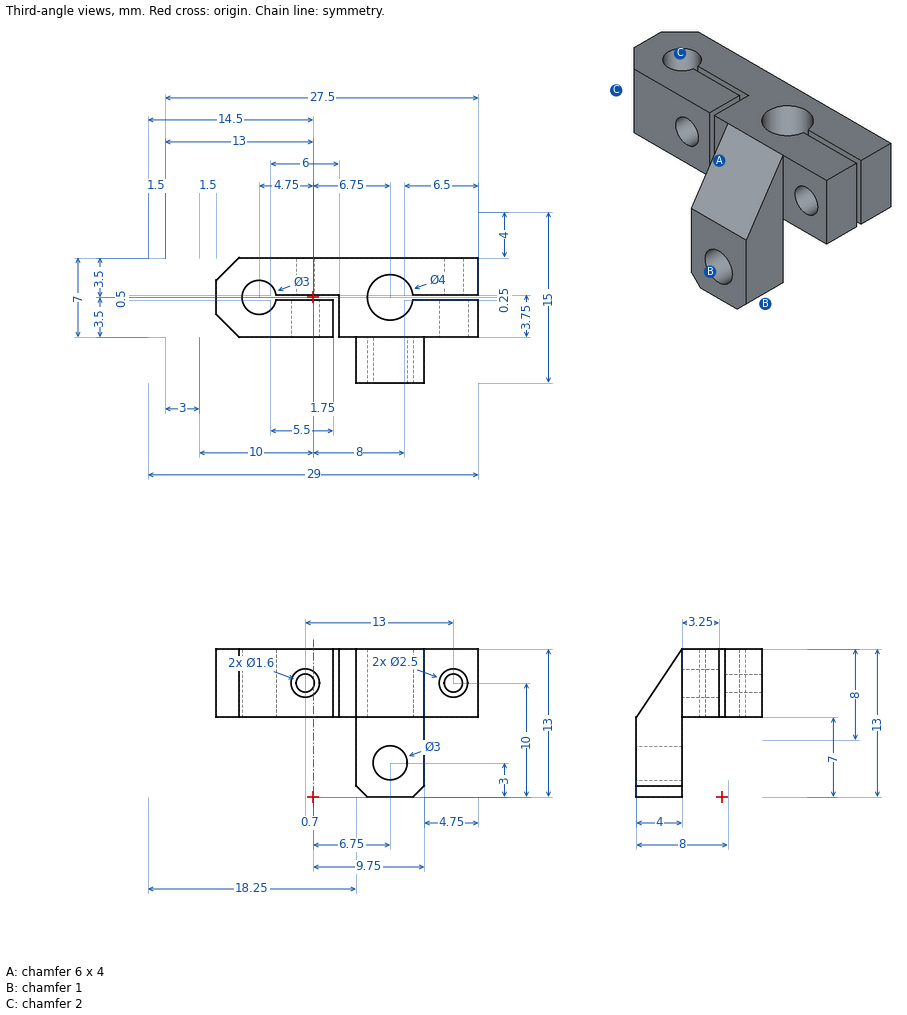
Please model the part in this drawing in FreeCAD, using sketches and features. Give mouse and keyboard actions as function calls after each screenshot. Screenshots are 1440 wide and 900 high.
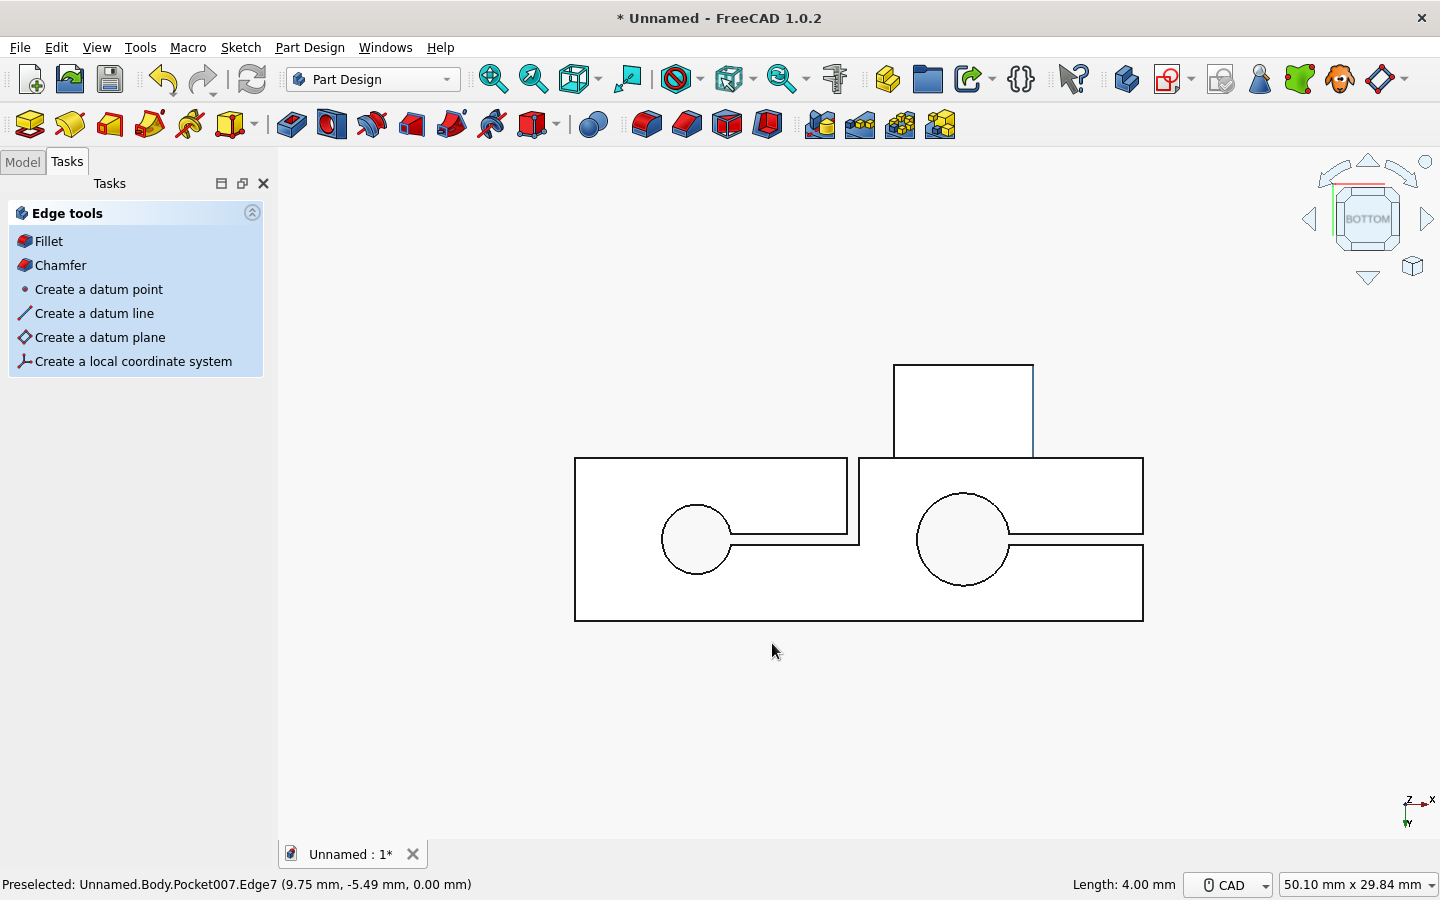
click(894, 392, ctrl)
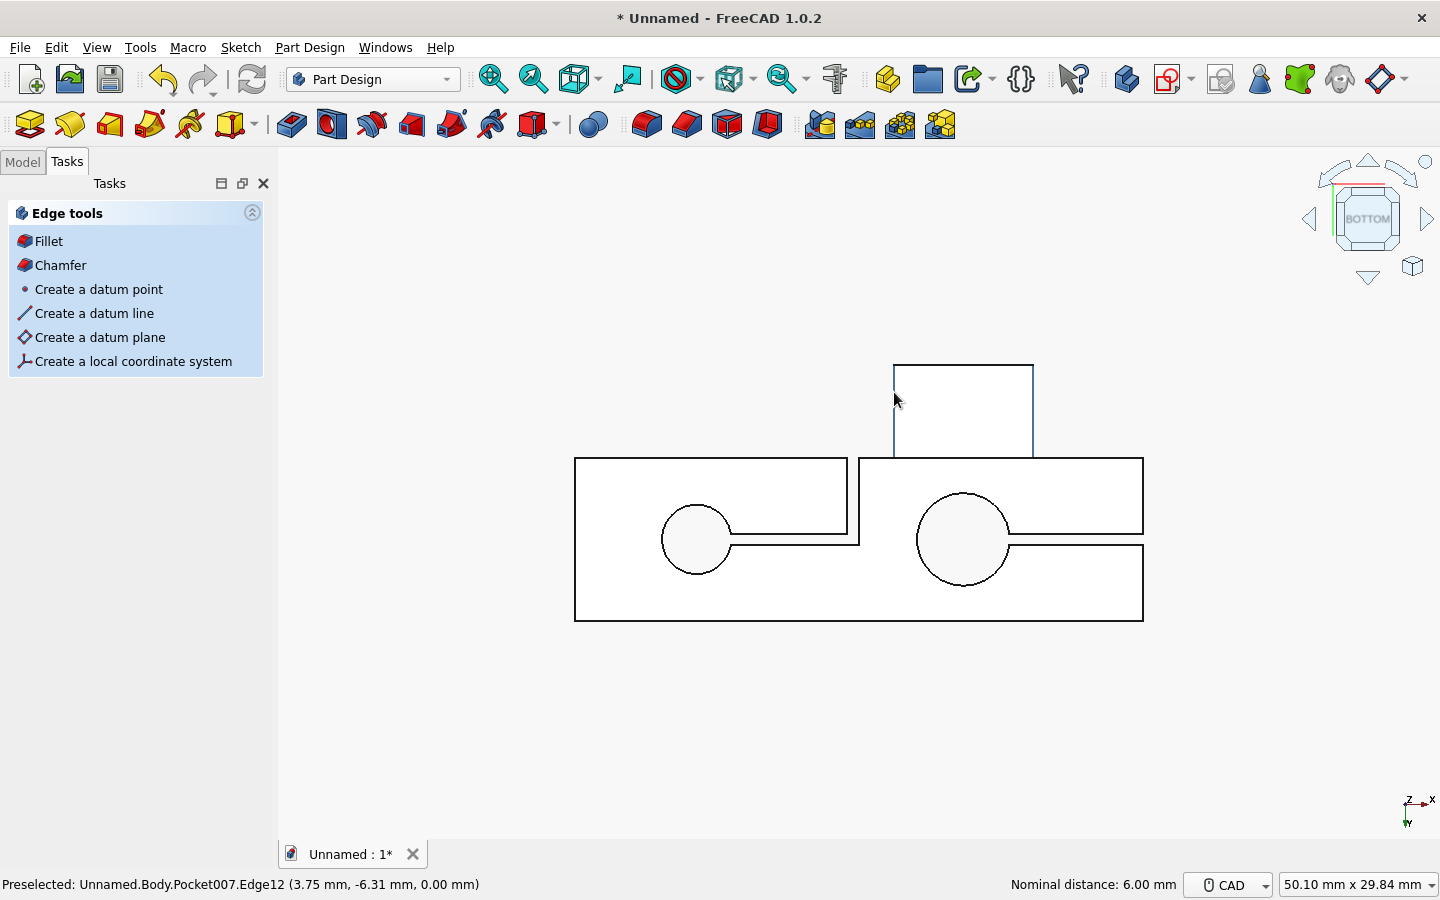
click(688, 124)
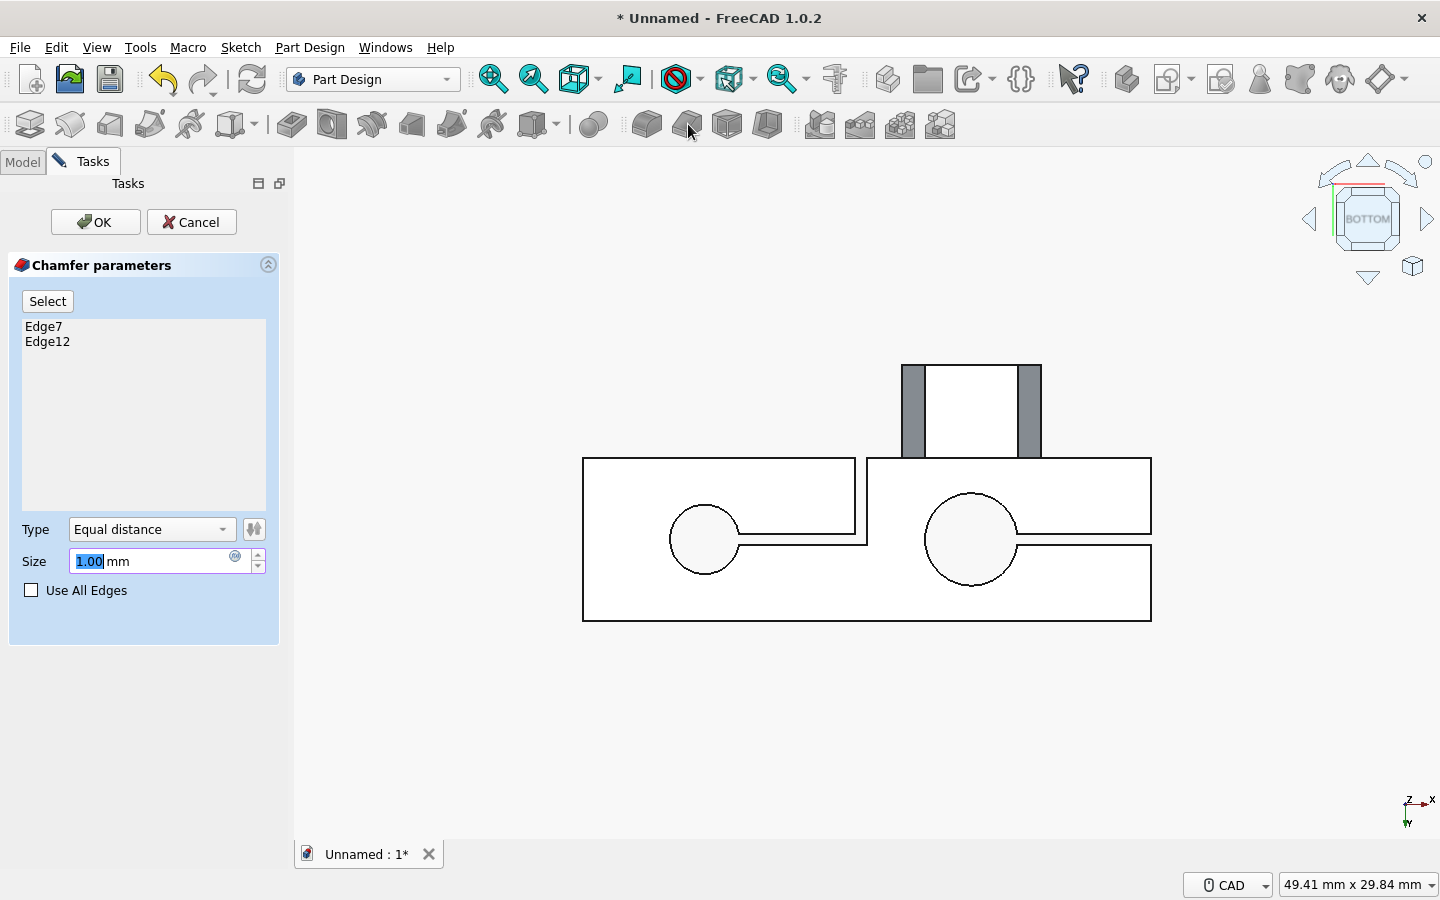
text(1)
key(Tab)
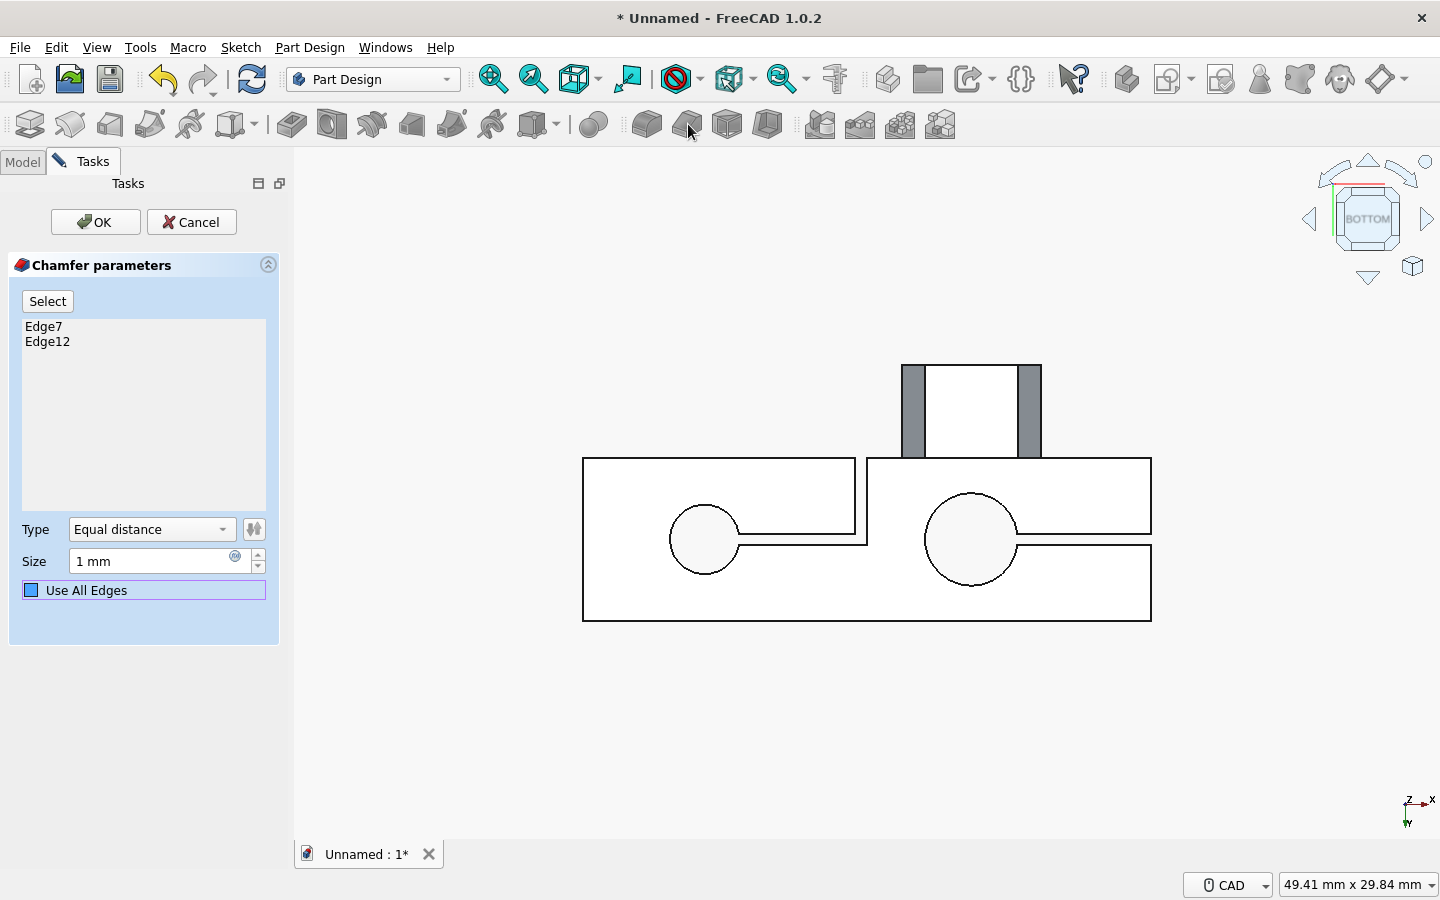
click(96, 222)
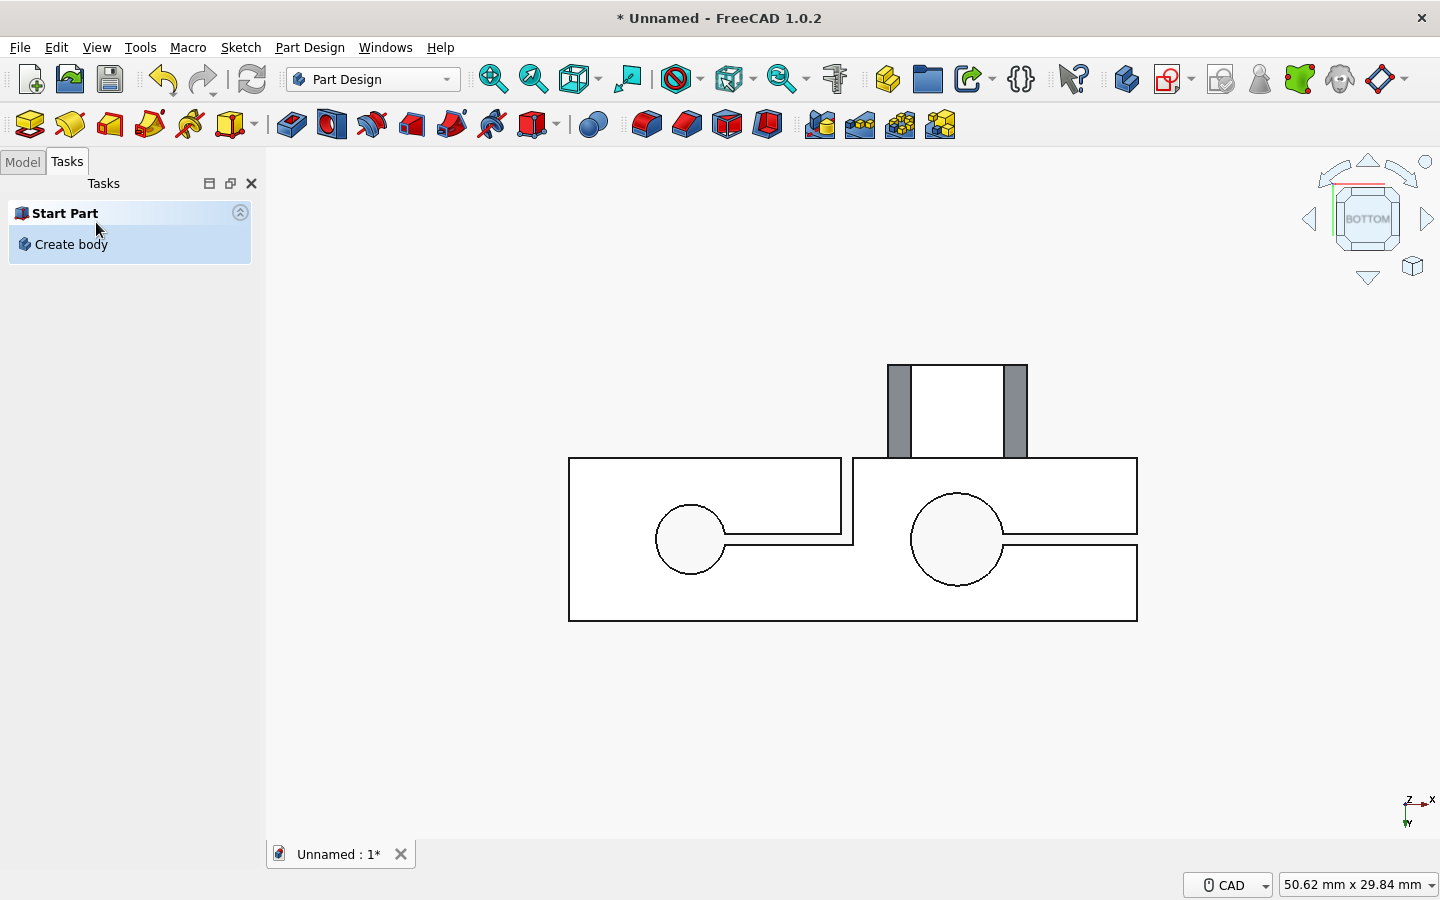
click(609, 562)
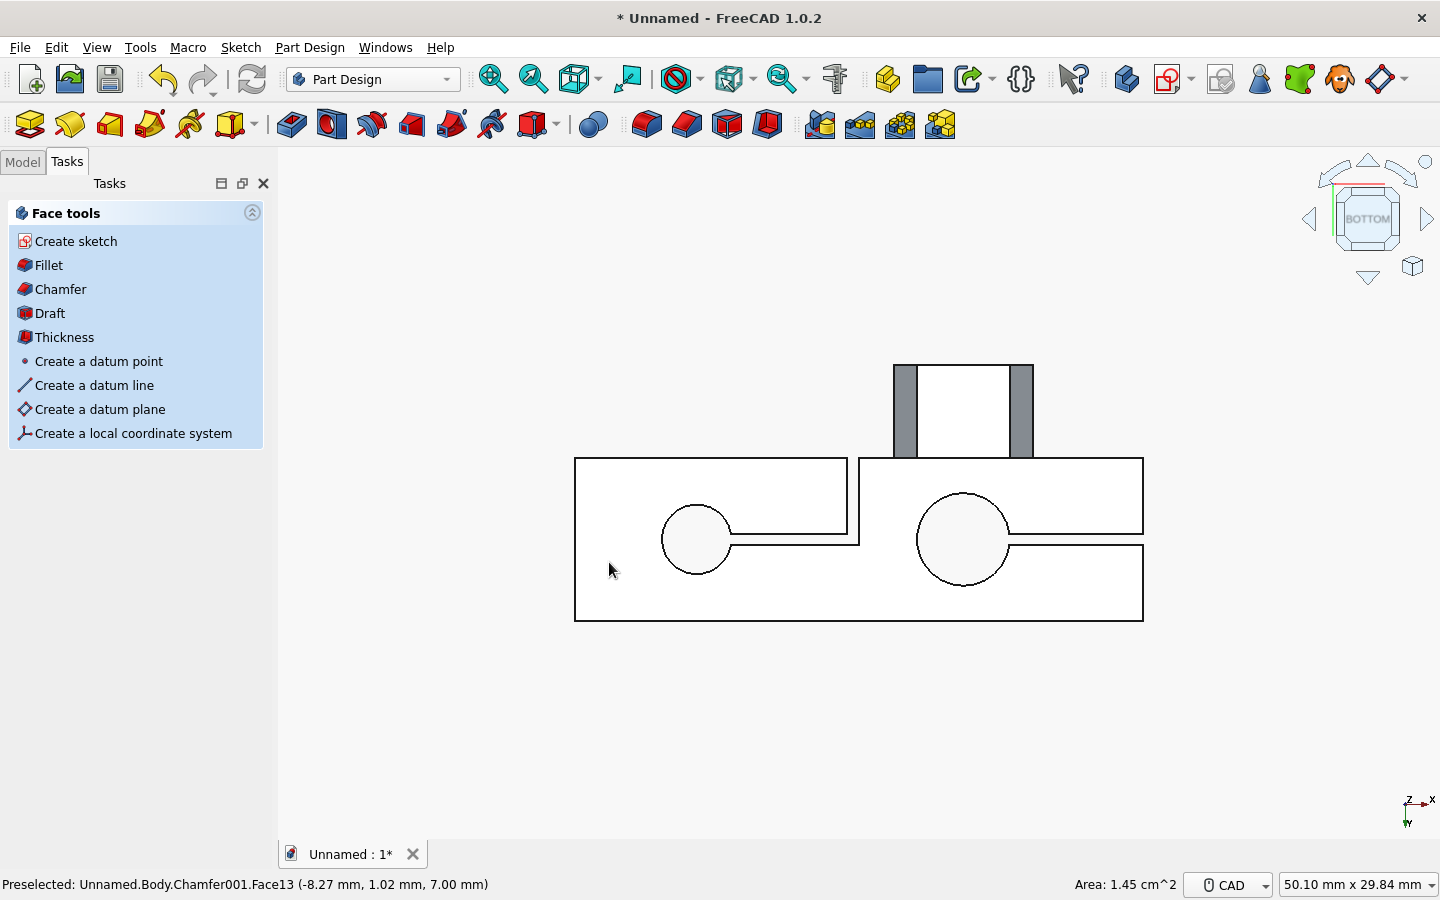
click(1168, 80)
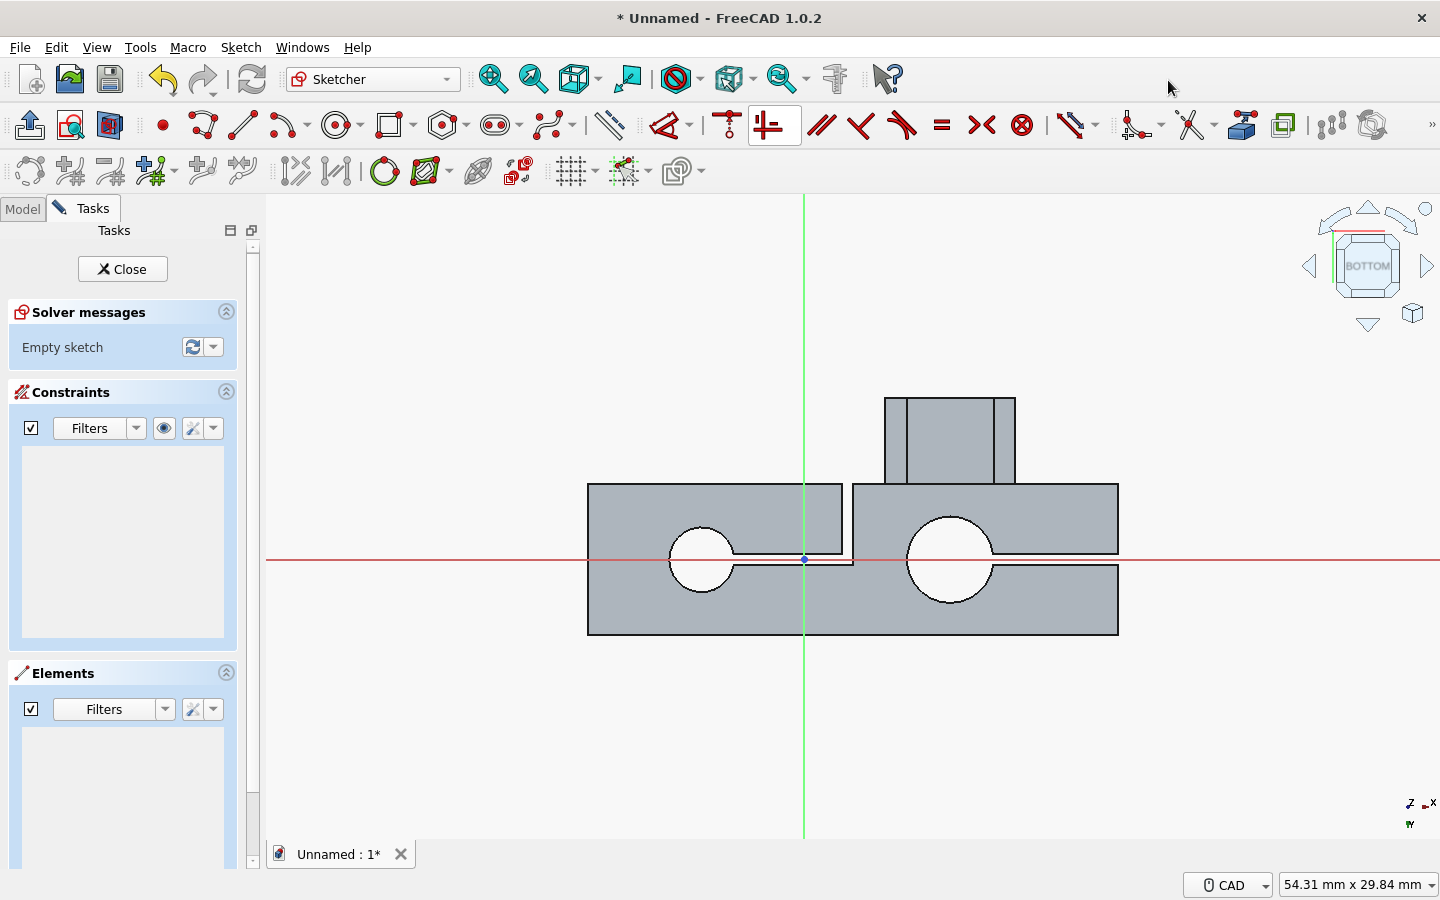
click(110, 126)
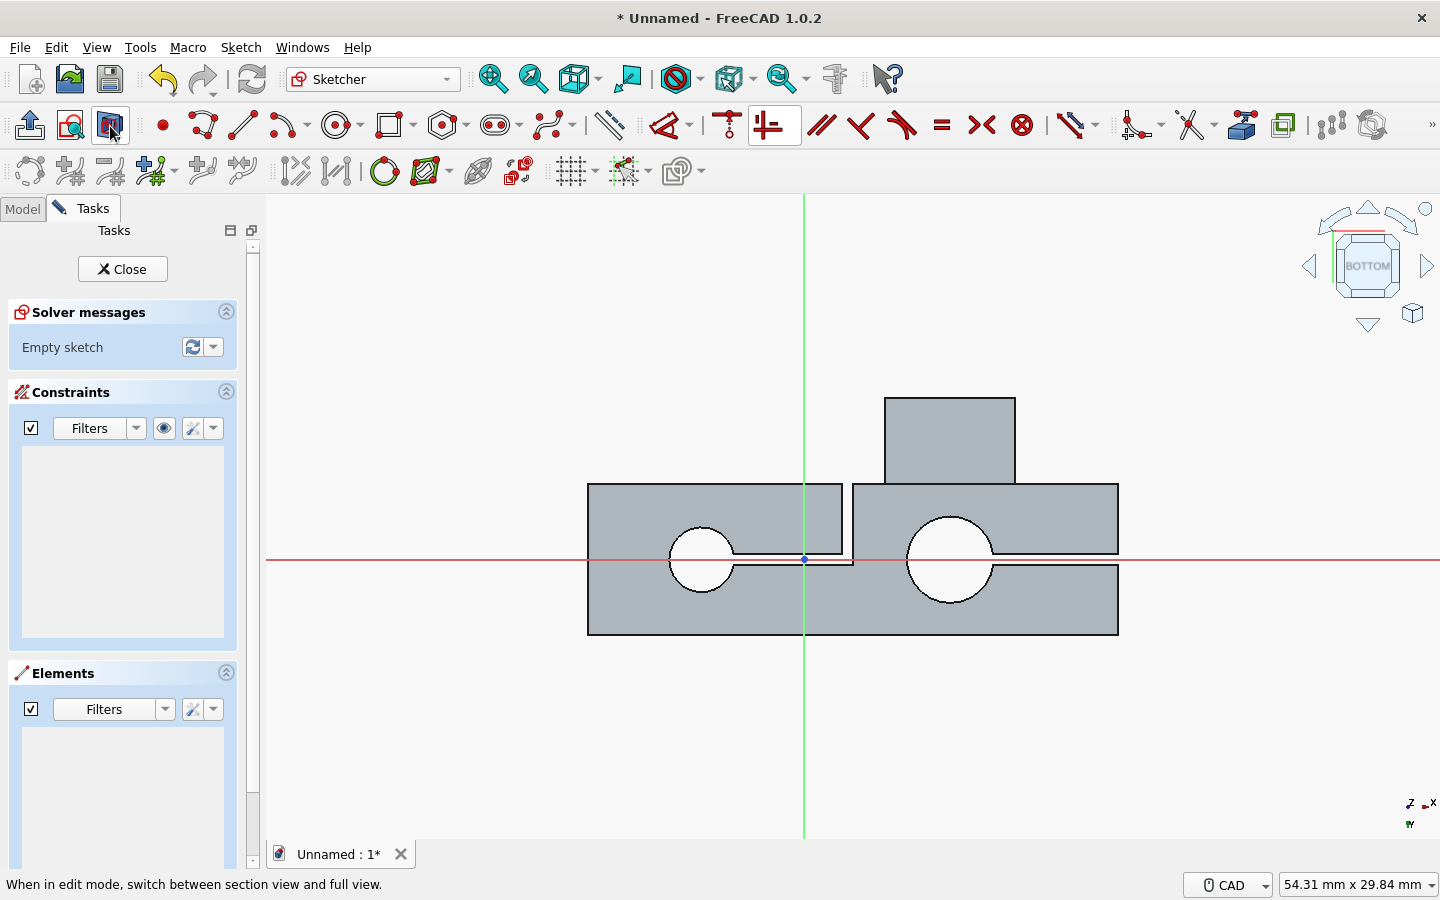
scroll(645, 585, up, 5)